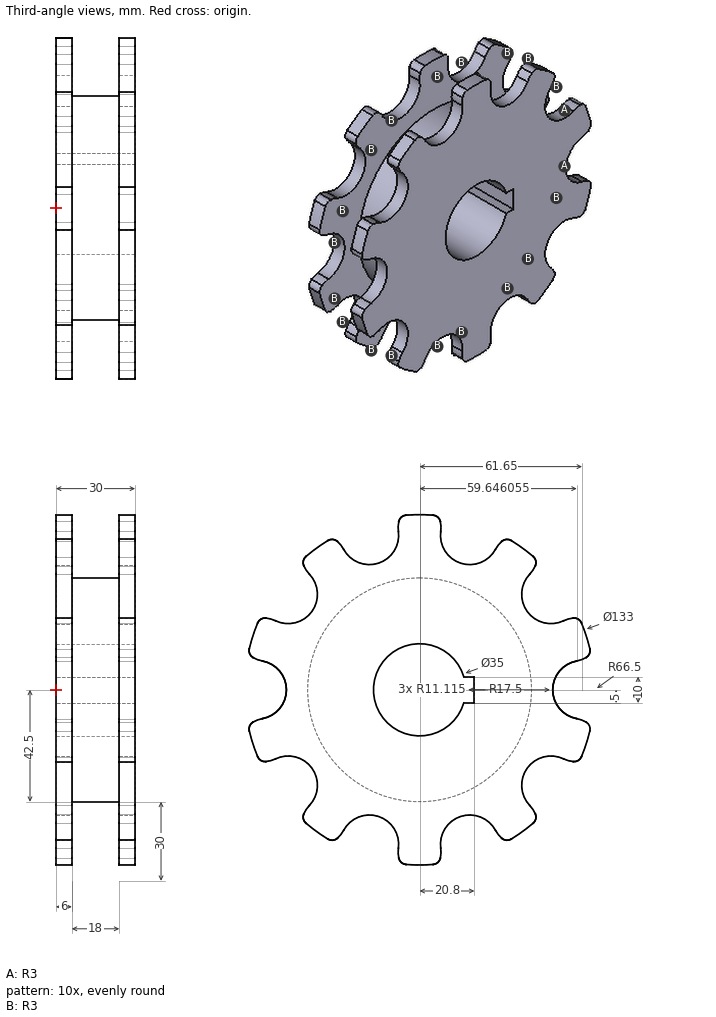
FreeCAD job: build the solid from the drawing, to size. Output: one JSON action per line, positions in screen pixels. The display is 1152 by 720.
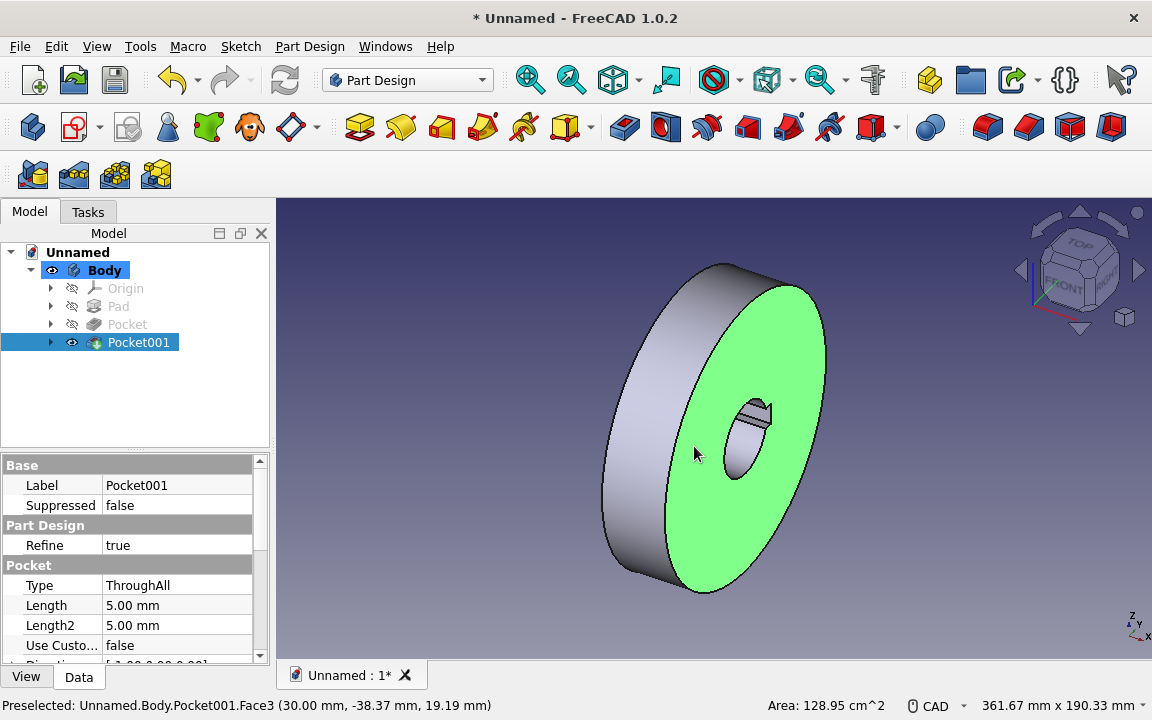
{"action": "left_click", "coordinate": [74, 128]}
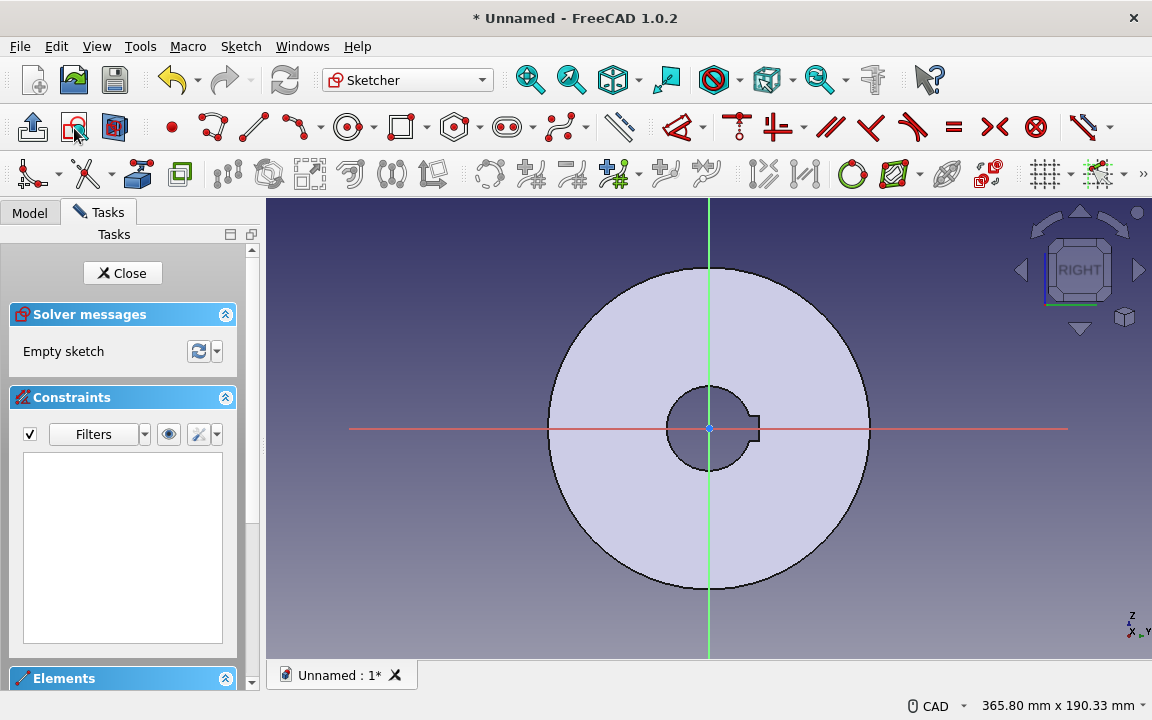
{"action": "scroll", "coordinate": [854, 428], "scroll_direction": "up", "scroll_amount": 6}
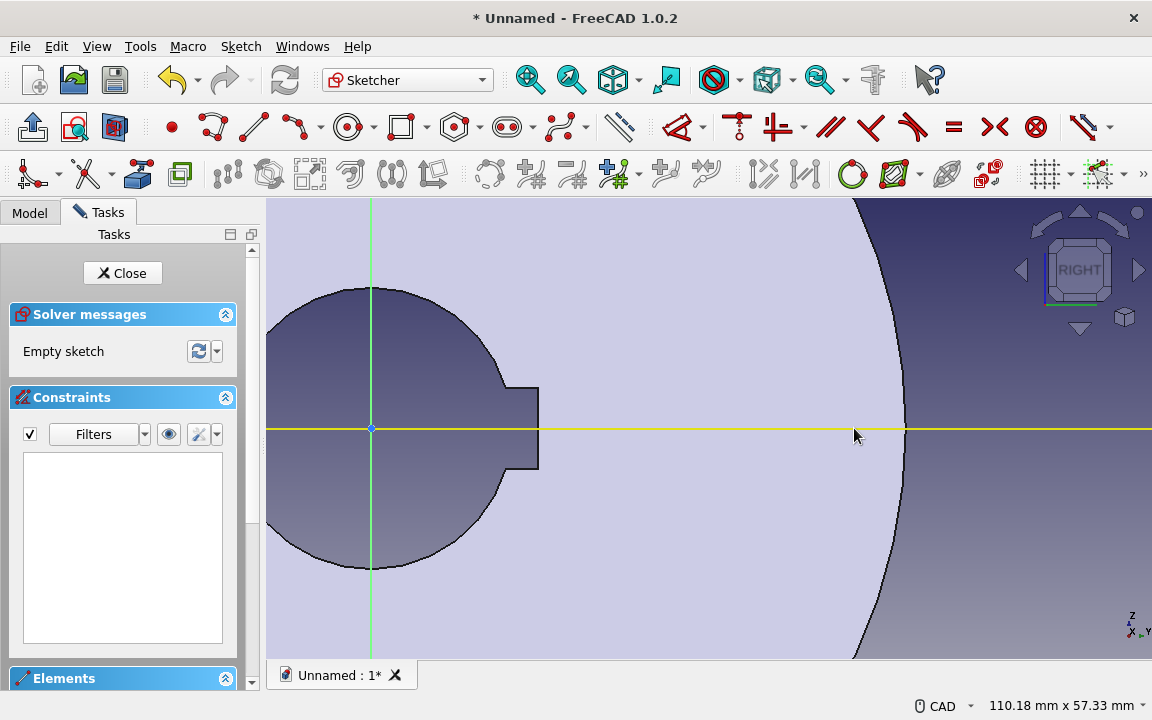
{"action": "left_click", "coordinate": [294, 128]}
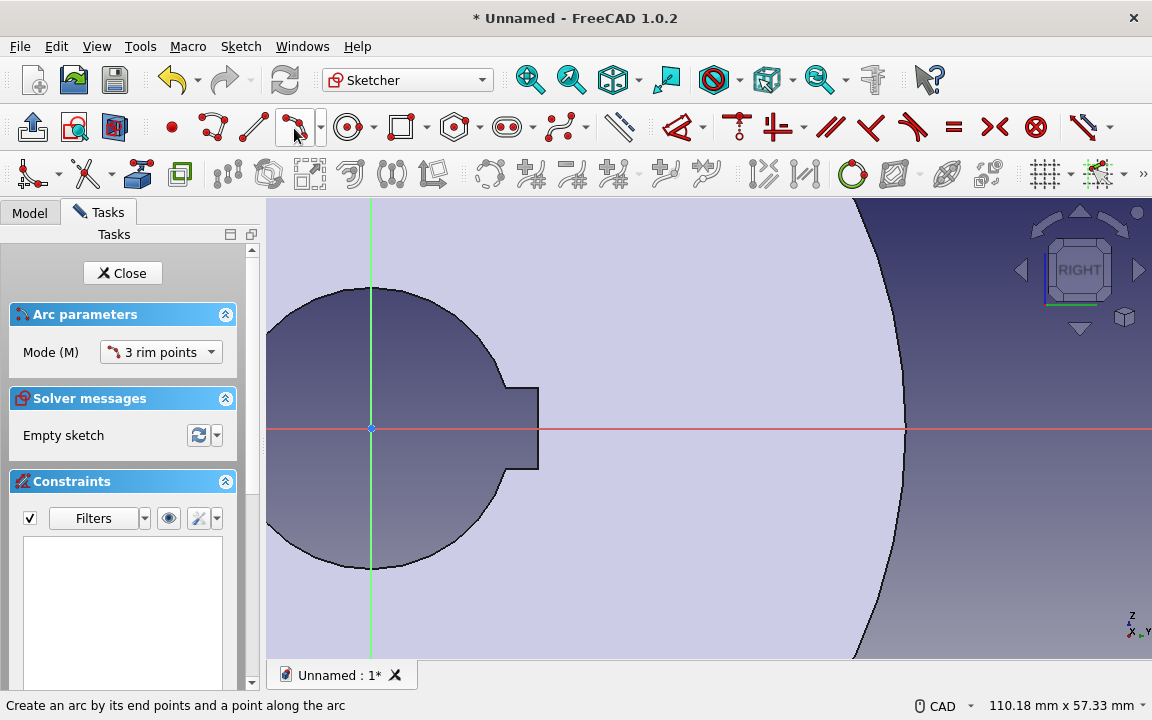
{"action": "left_click", "coordinate": [851, 341]}
{"action": "left_click", "coordinate": [851, 516]}
{"action": "left_click", "coordinate": [781, 404]}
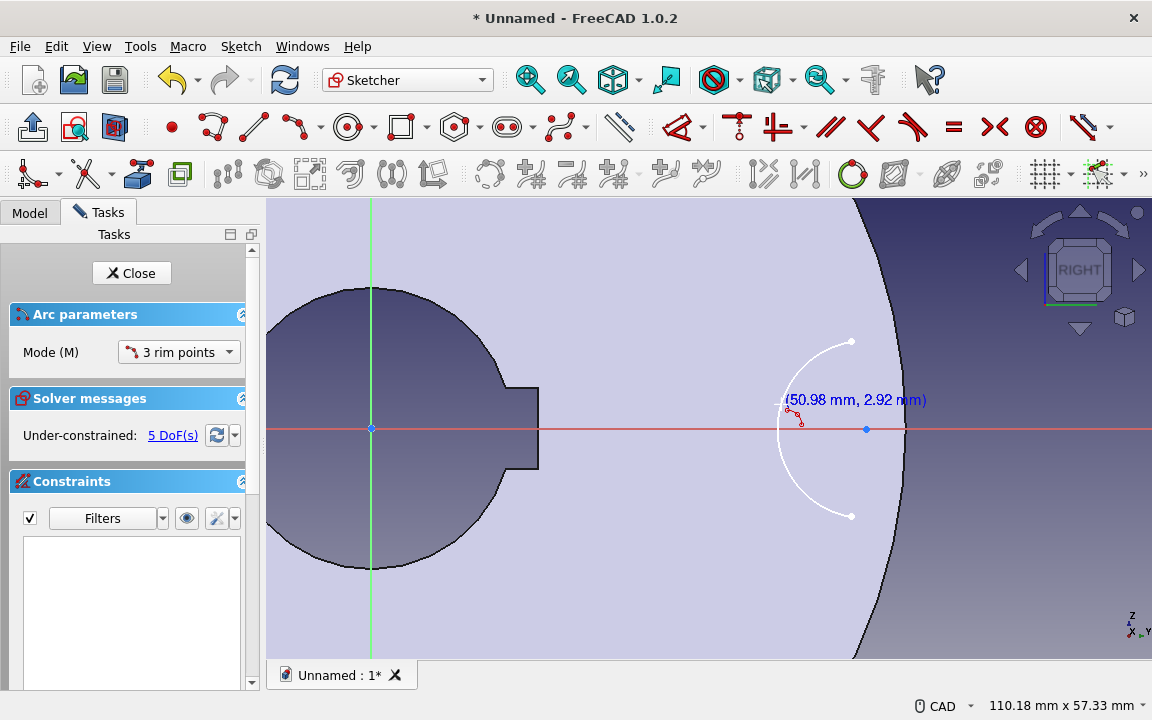
{"action": "left_click", "coordinate": [851, 517]}
{"action": "left_click", "coordinate": [894, 538]}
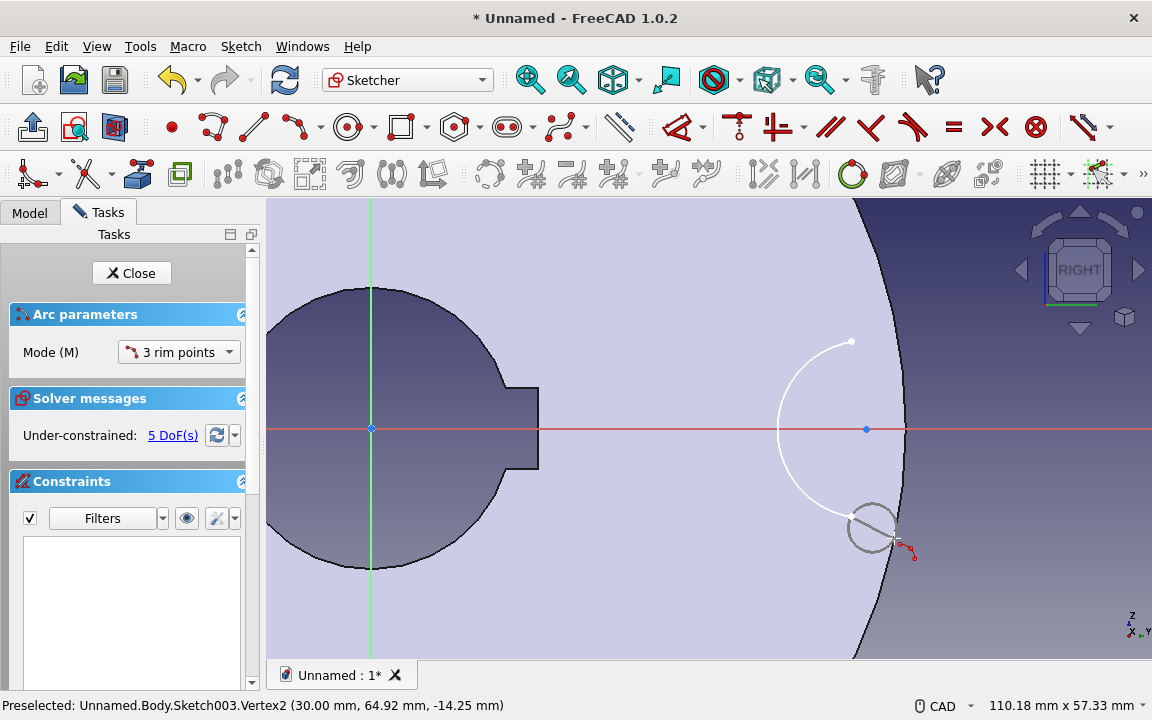
{"action": "scroll", "coordinate": [874, 524], "scroll_direction": "up", "scroll_amount": 8}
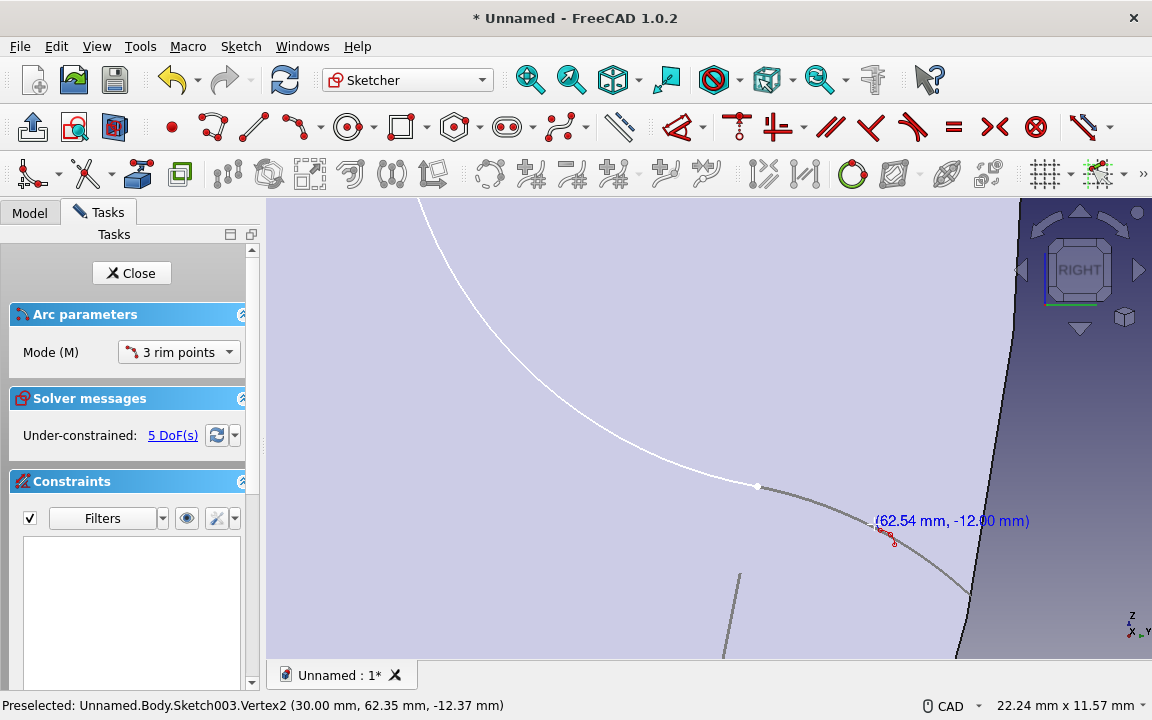
{"action": "left_click", "coordinate": [872, 522]}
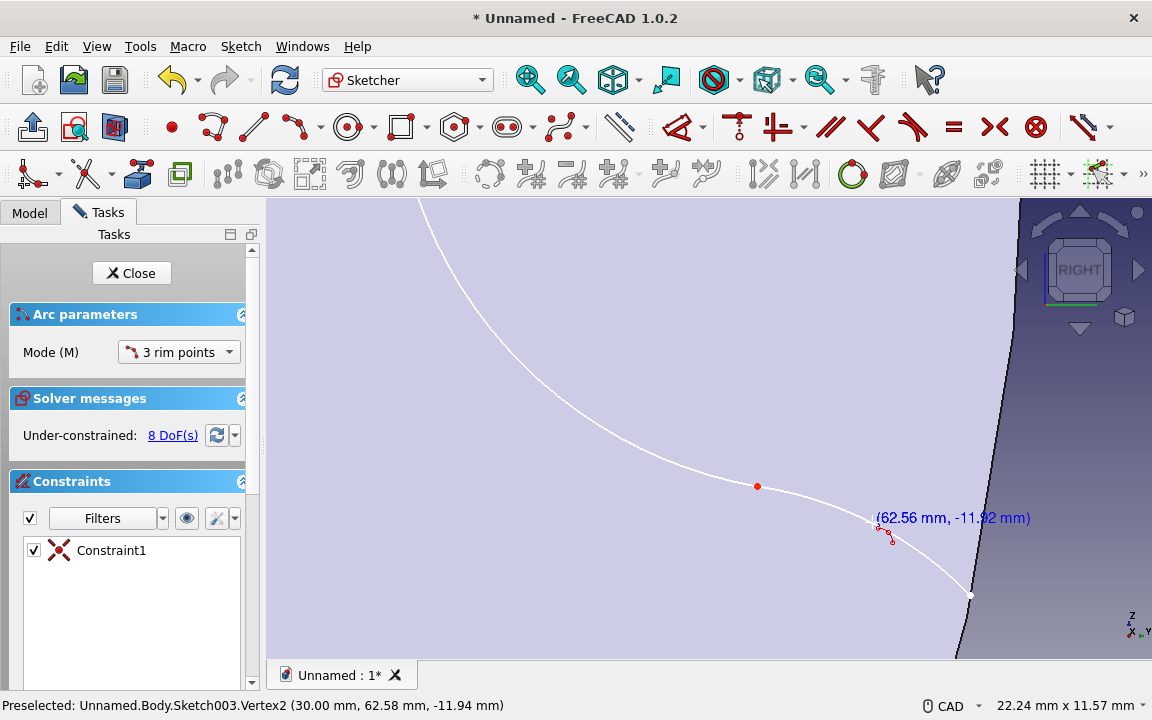
{"action": "scroll", "coordinate": [877, 525], "scroll_direction": "down", "scroll_amount": 8}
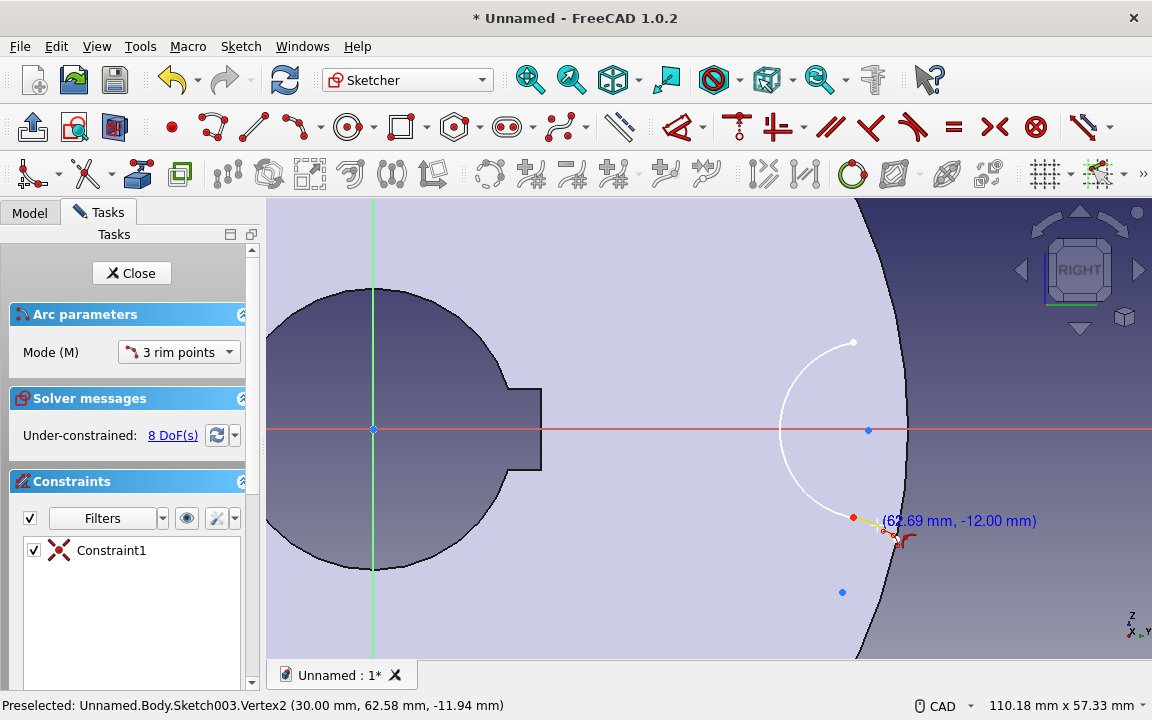
{"action": "left_click", "coordinate": [896, 540]}
{"action": "left_click", "coordinate": [897, 320]}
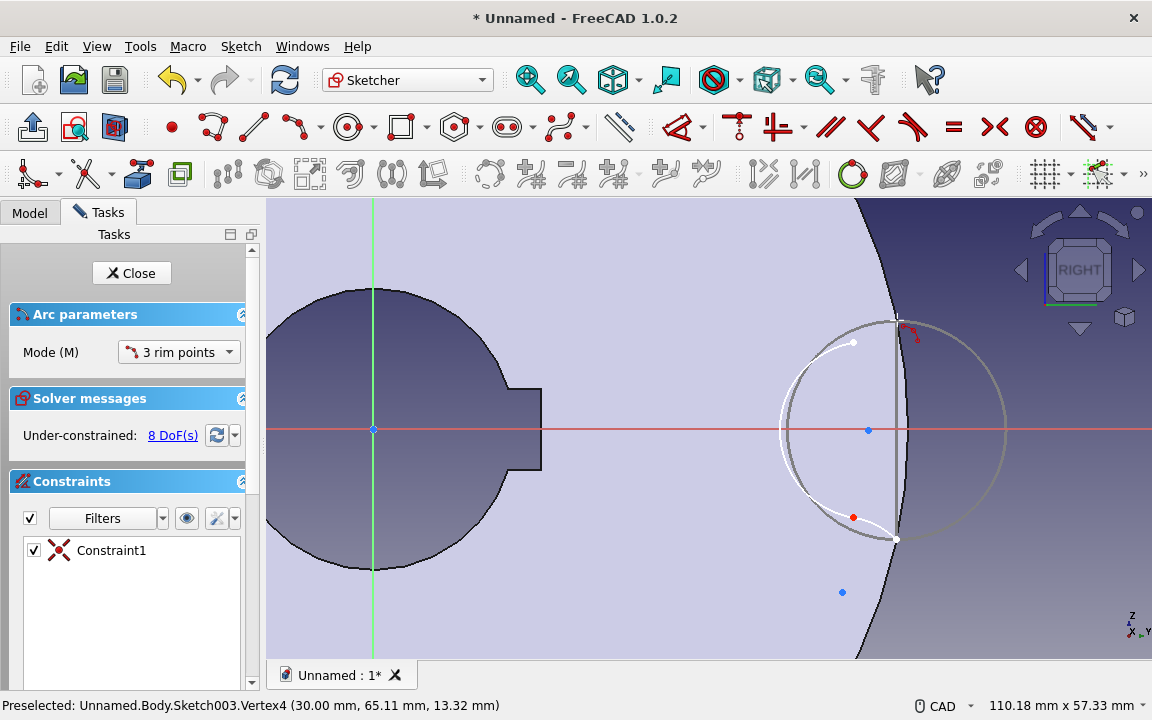
{"action": "scroll", "coordinate": [908, 451], "scroll_direction": "up", "scroll_amount": 2}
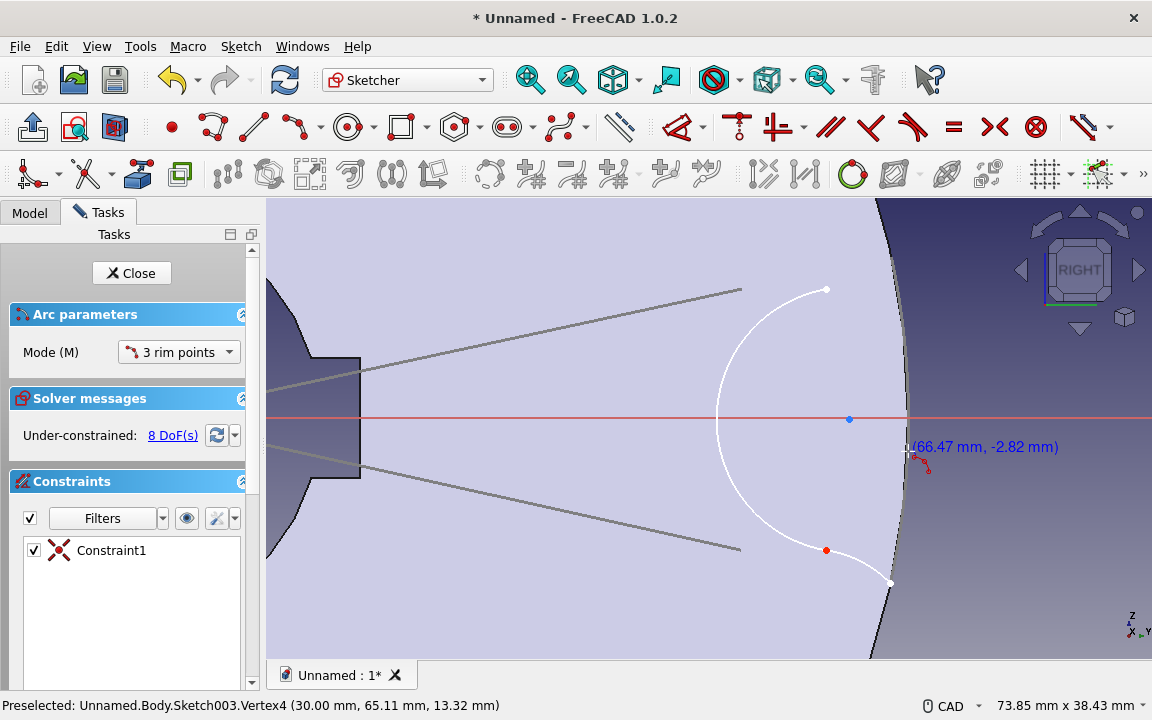
{"action": "left_click", "coordinate": [907, 451]}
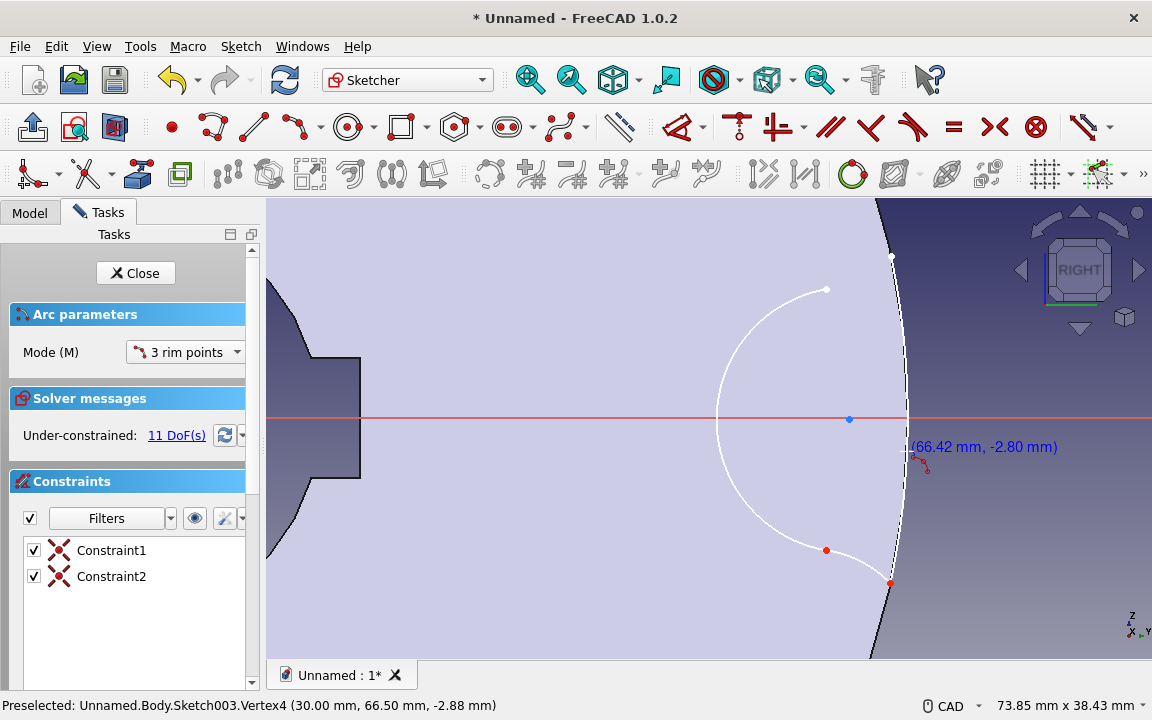
{"action": "left_click", "coordinate": [891, 257]}
{"action": "left_click", "coordinate": [826, 289]}